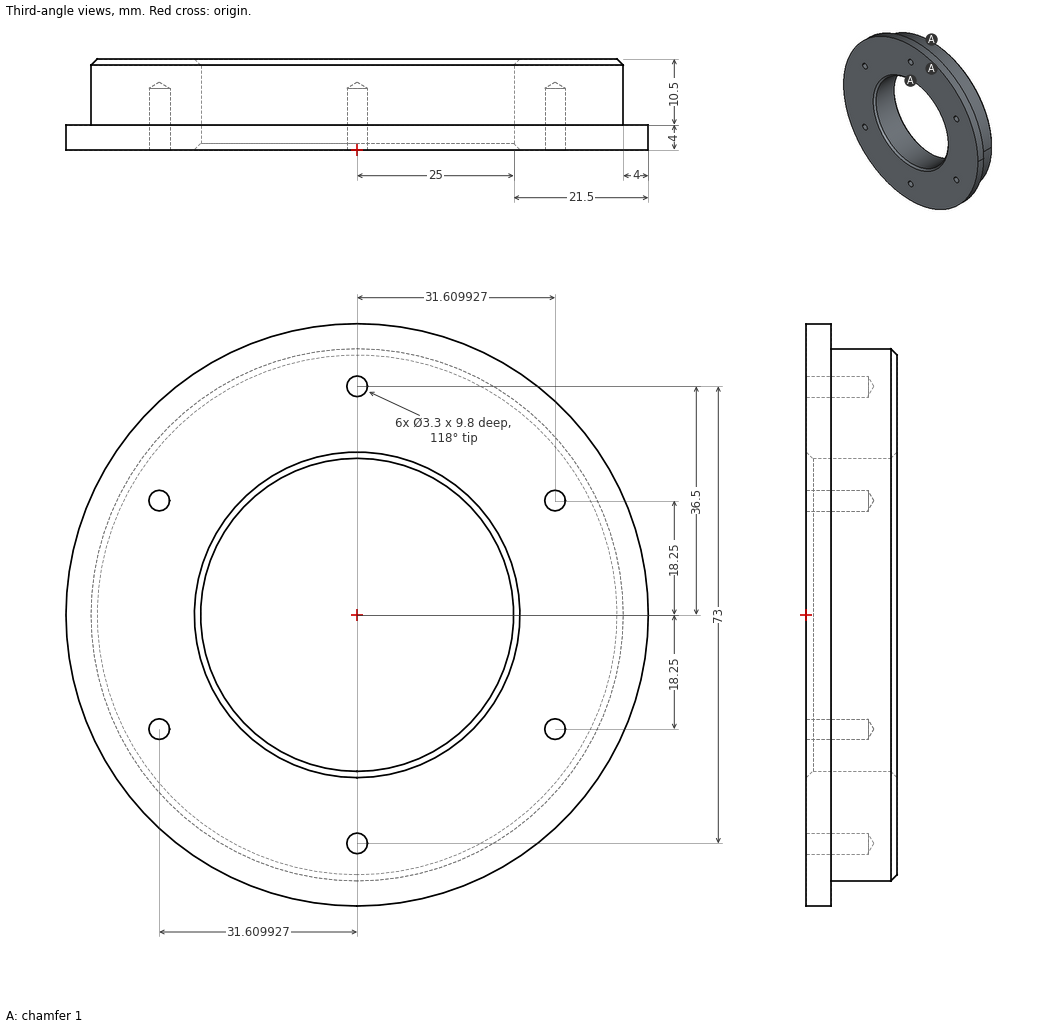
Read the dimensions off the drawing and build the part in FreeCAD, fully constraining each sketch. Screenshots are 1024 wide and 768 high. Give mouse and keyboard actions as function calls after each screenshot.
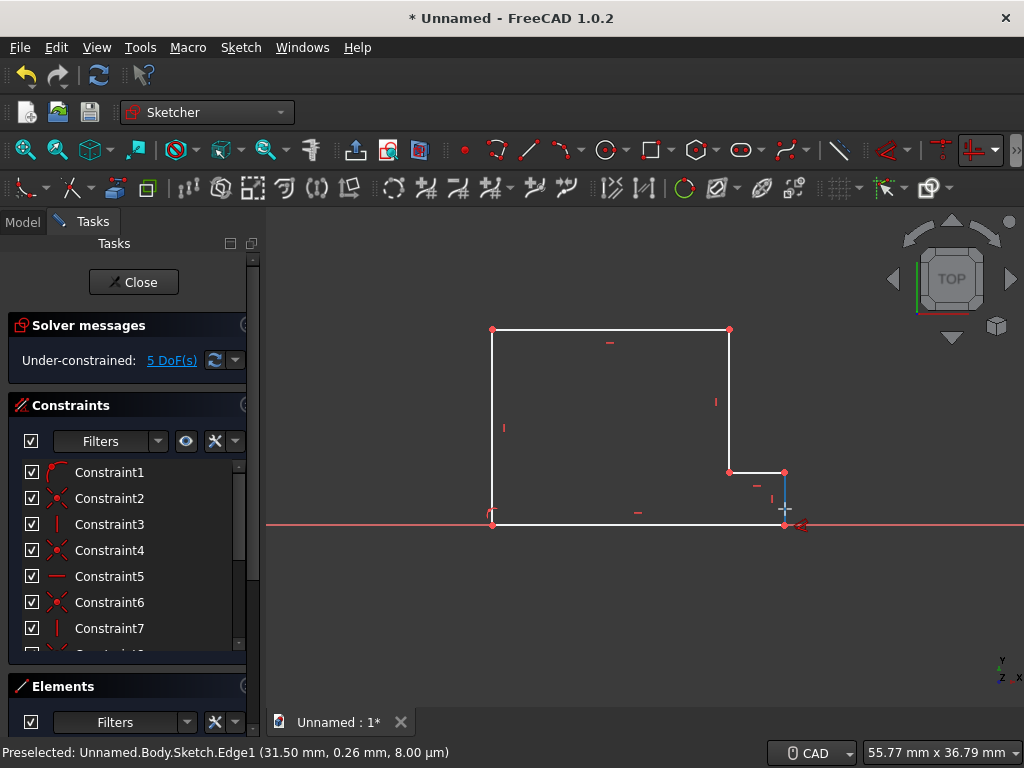
click(785, 509)
click(819, 499)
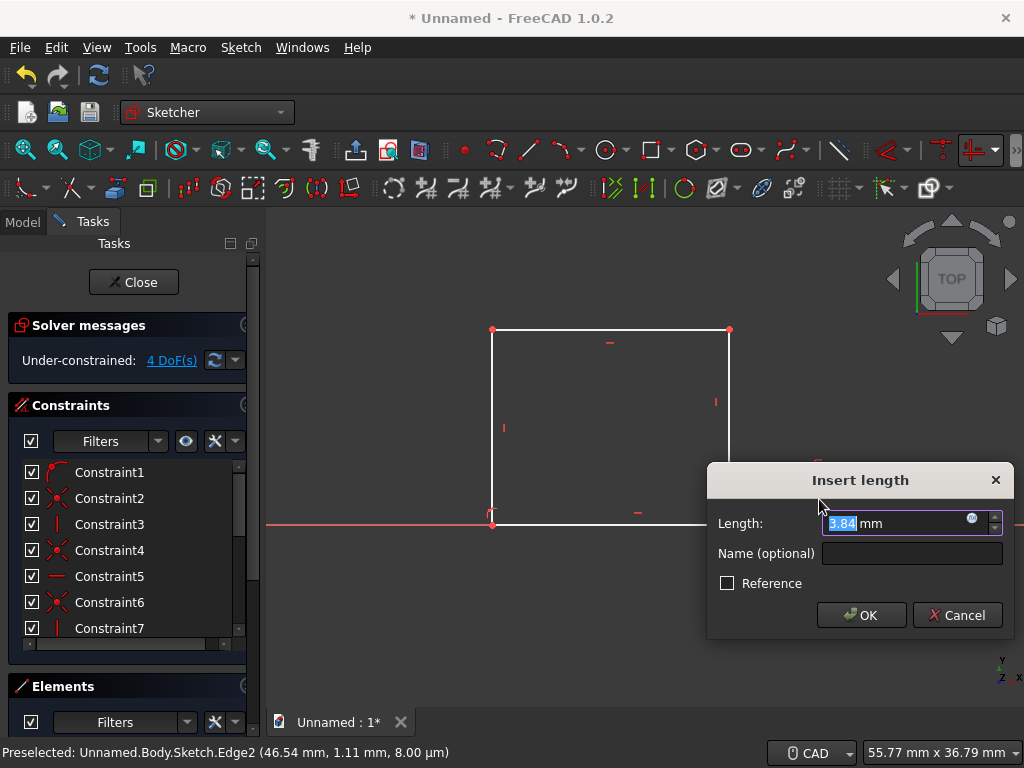
text(4)
key(Return)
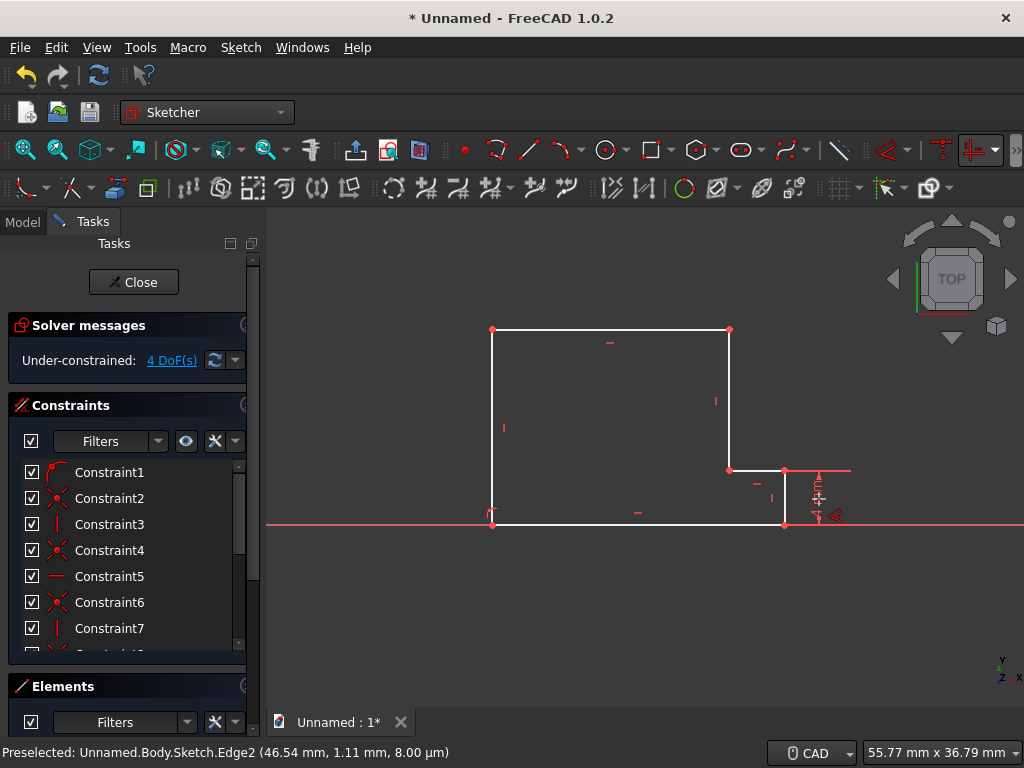
click(768, 471)
click(744, 505)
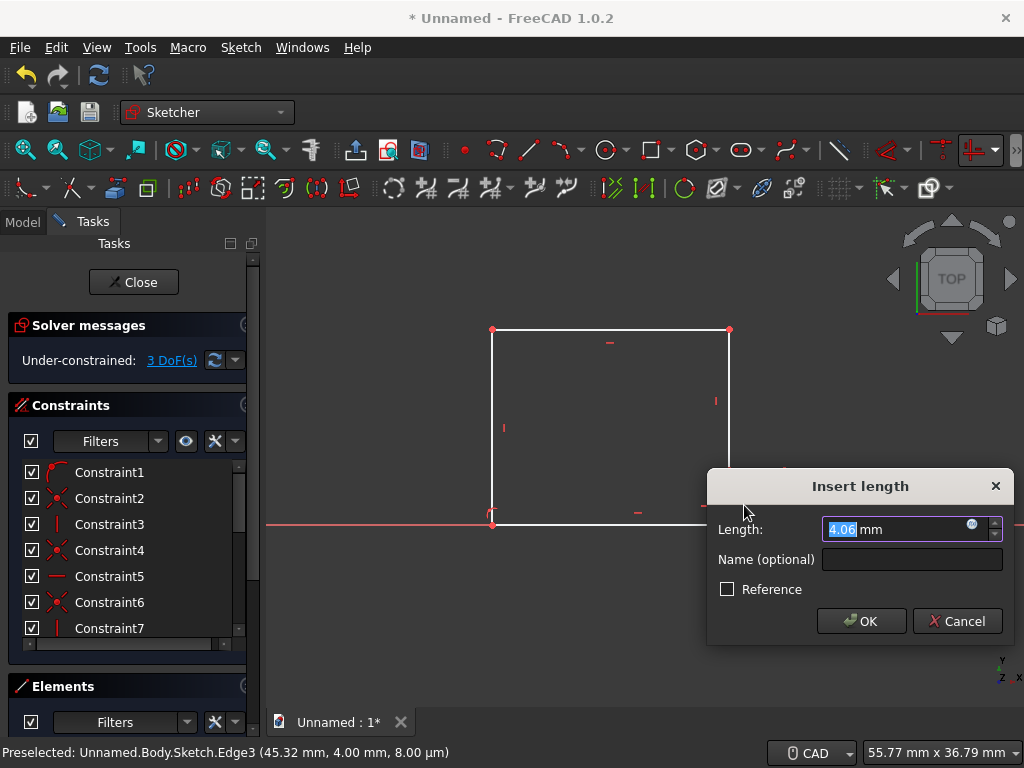
text(4)
key(Return)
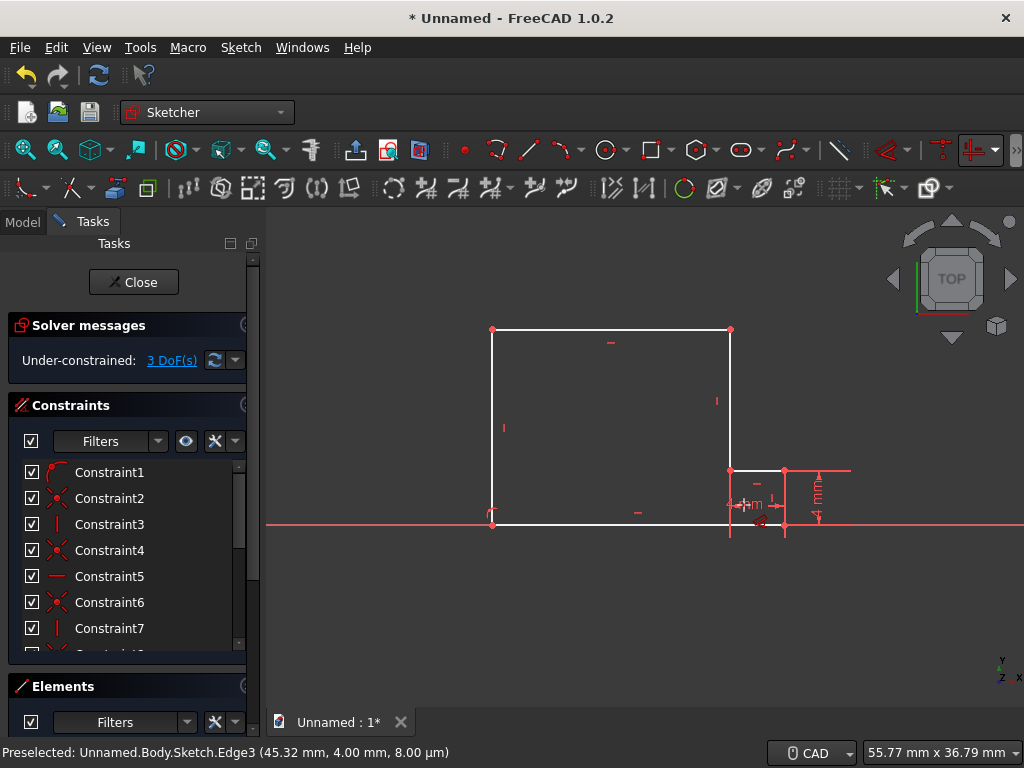
click(492, 525)
click(393, 559)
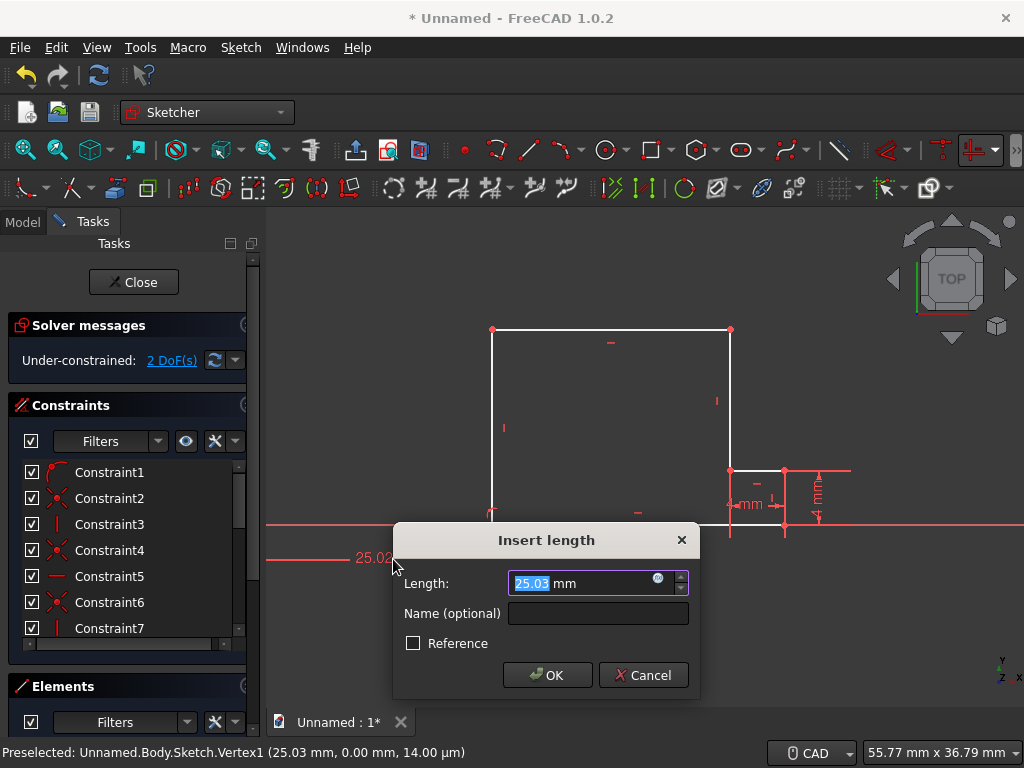
text(25)
key(Return)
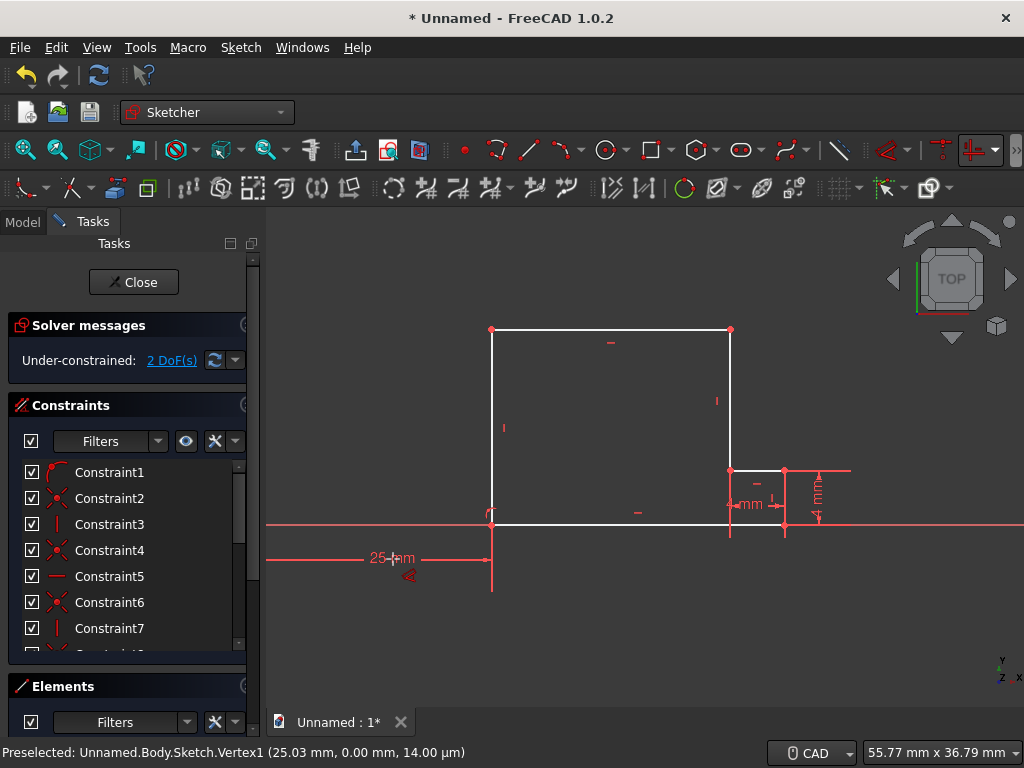
click(580, 525)
click(638, 559)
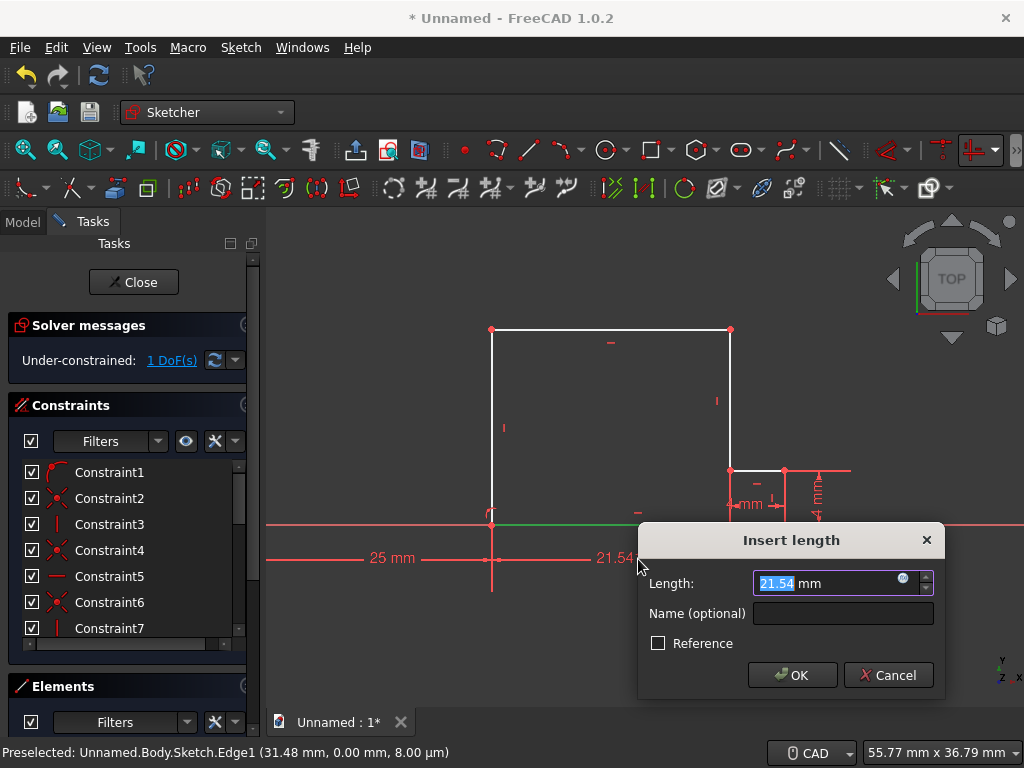
text(21.5)
key(Return)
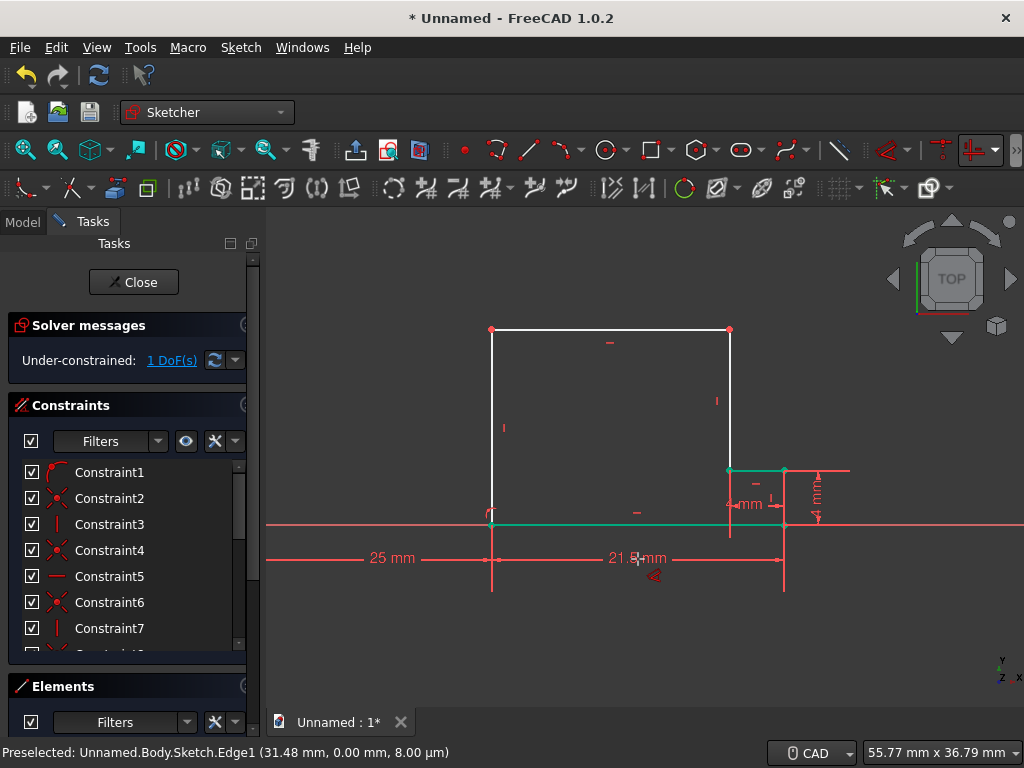
click(730, 428)
click(764, 400)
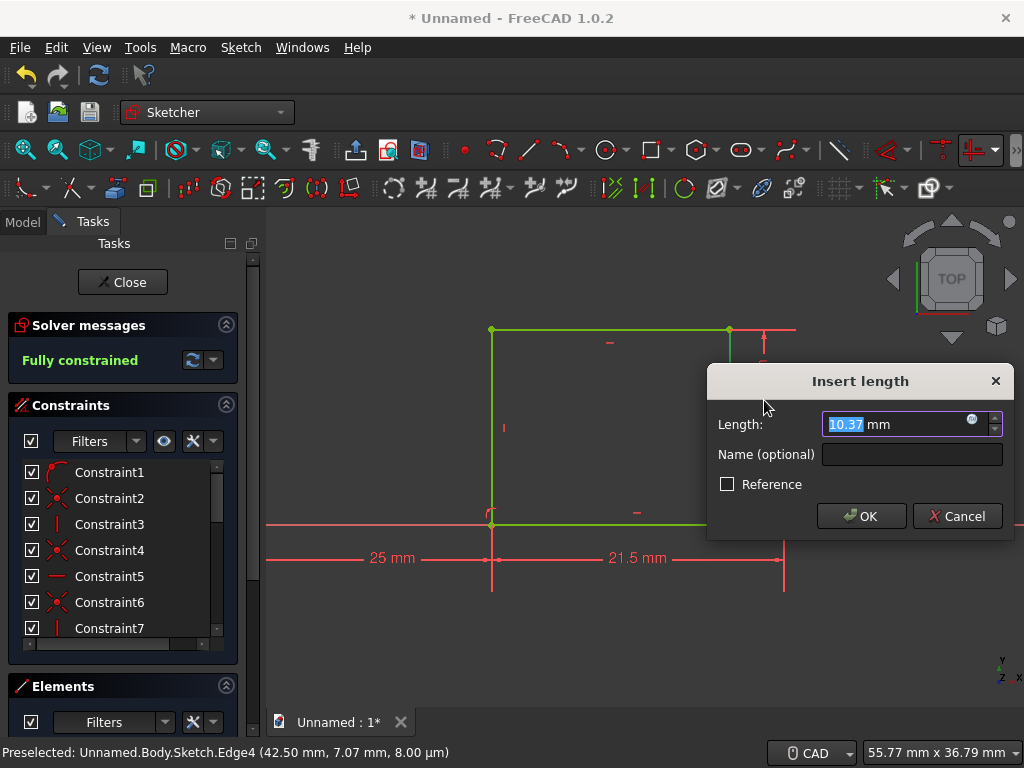
text(10.5)
key(Return)
key(Escape)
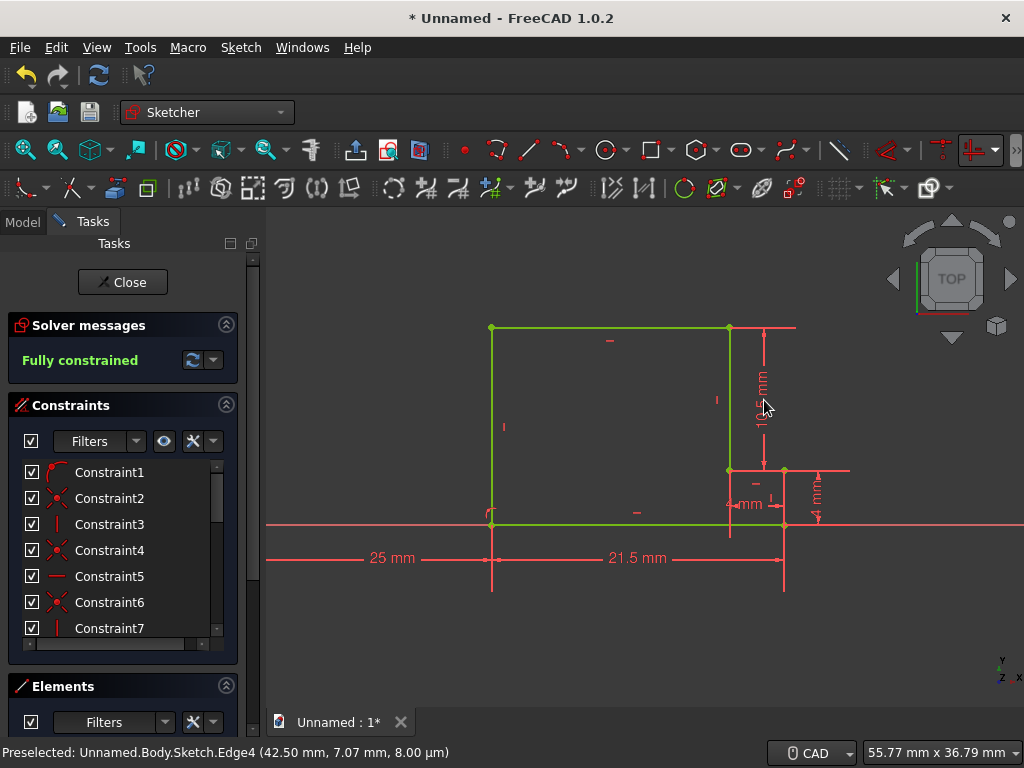
click(123, 282)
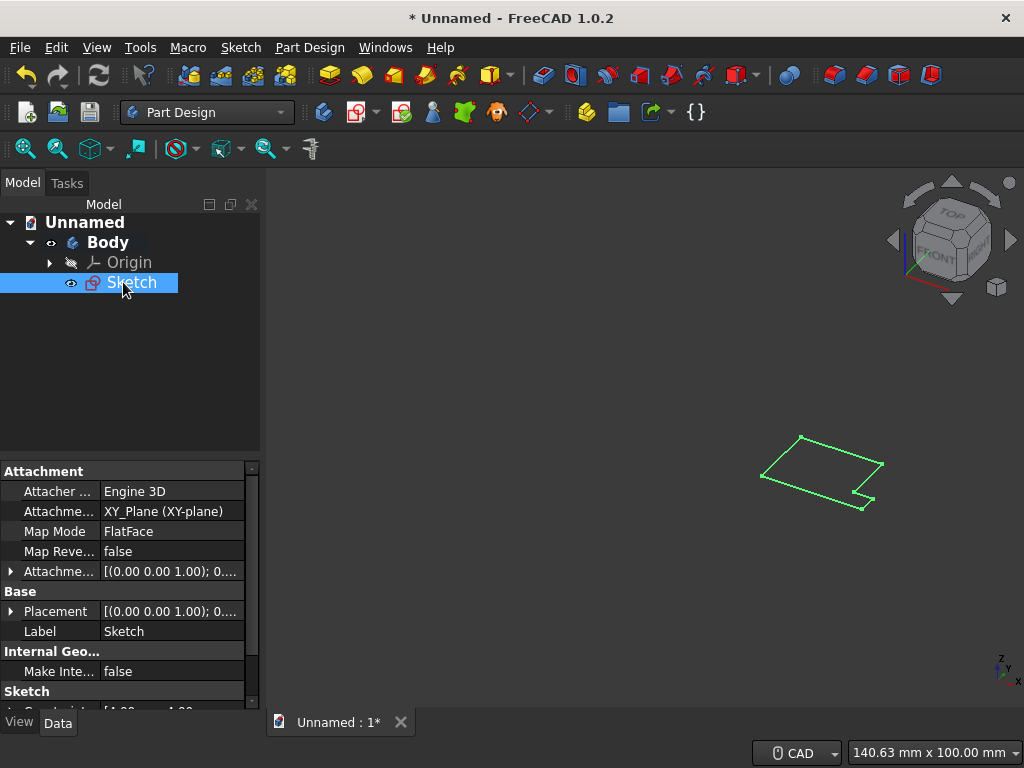
click(362, 76)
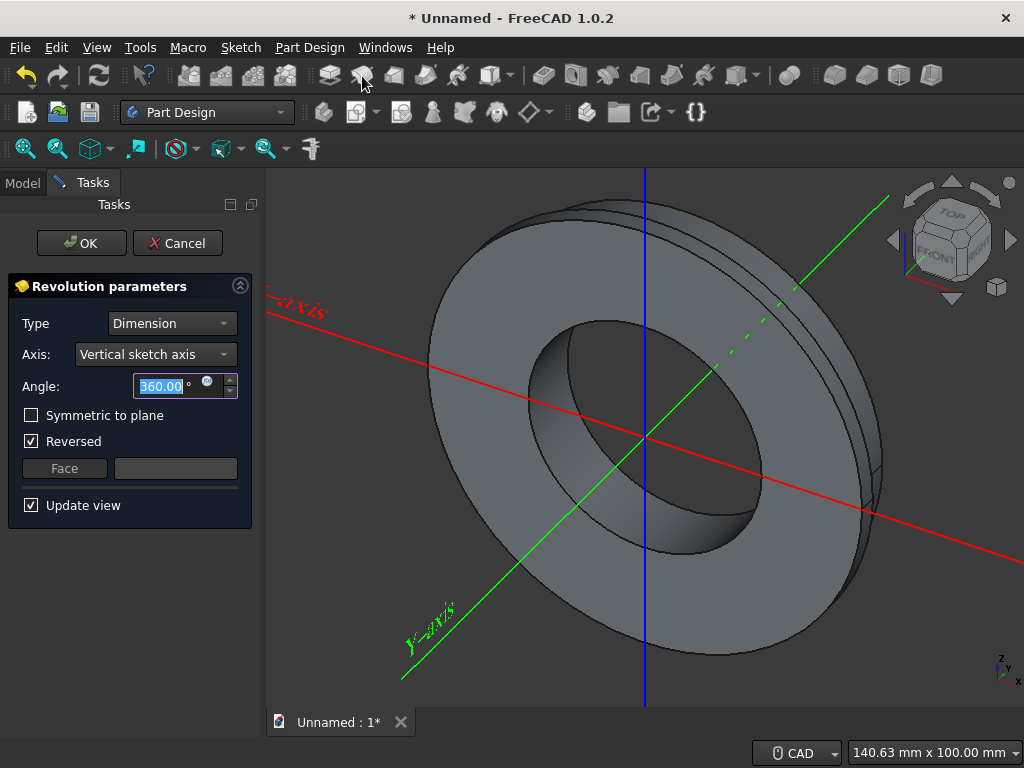
click(82, 243)